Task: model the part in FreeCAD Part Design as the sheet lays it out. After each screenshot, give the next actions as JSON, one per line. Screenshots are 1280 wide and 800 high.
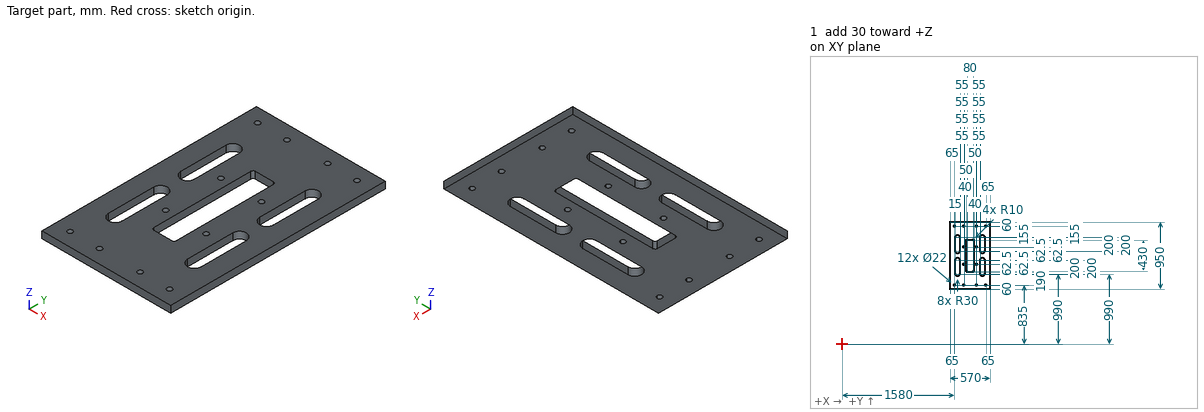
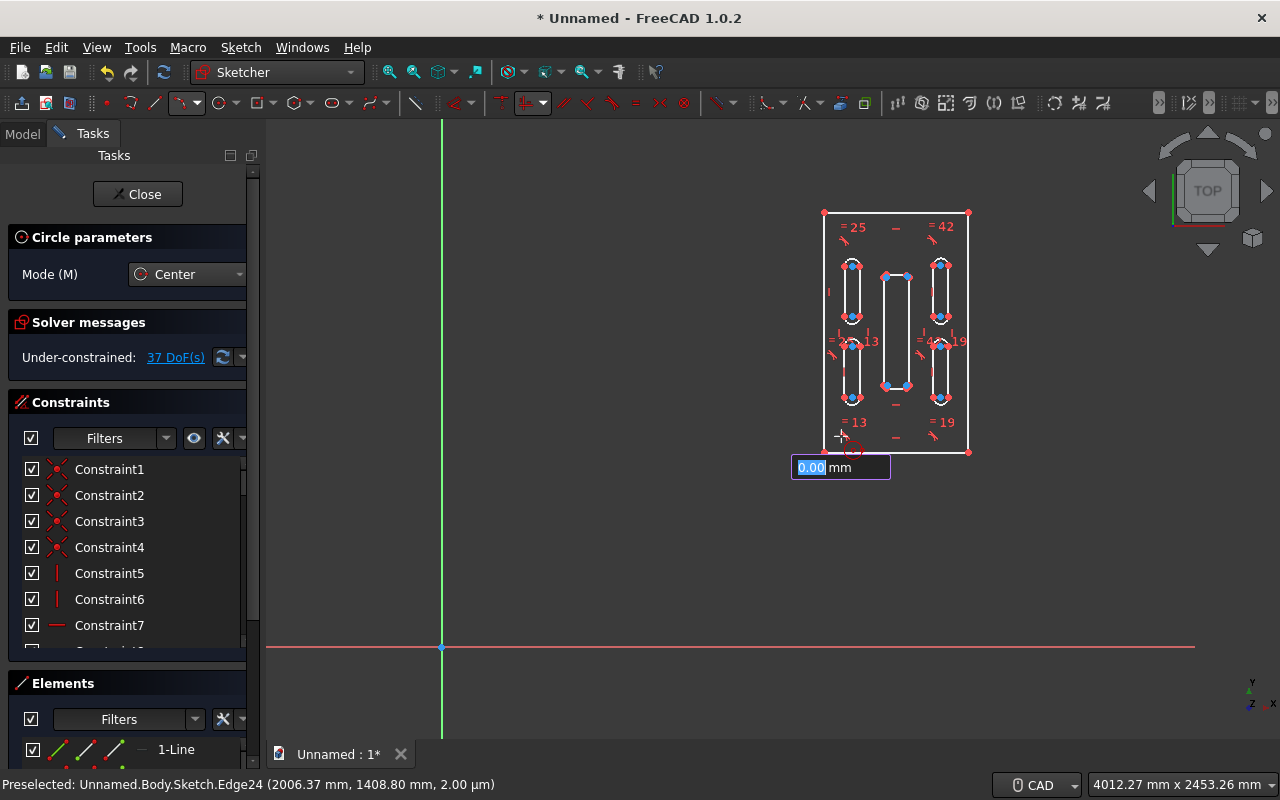
{"action": "scroll", "coordinate": [843, 434], "scroll_direction": "up", "scroll_amount": 9}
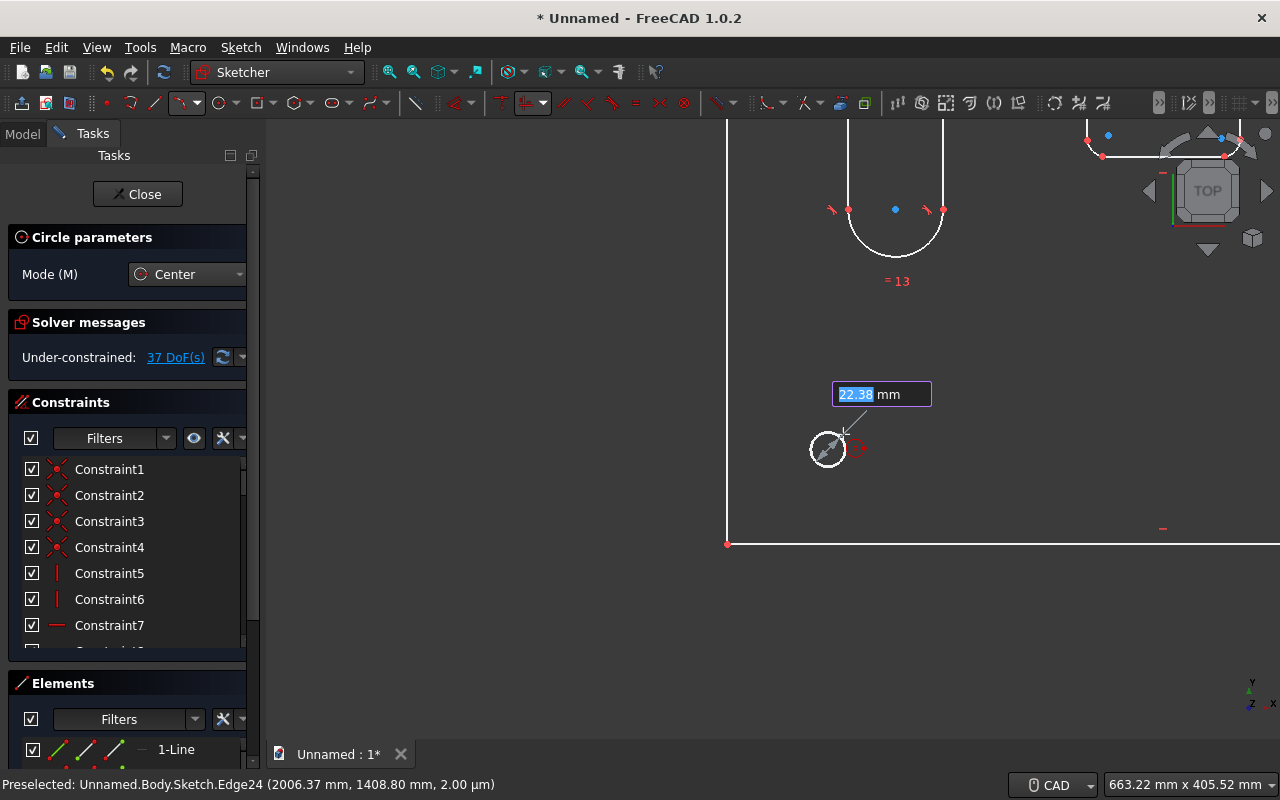
{"action": "left_click", "coordinate": [840, 433]}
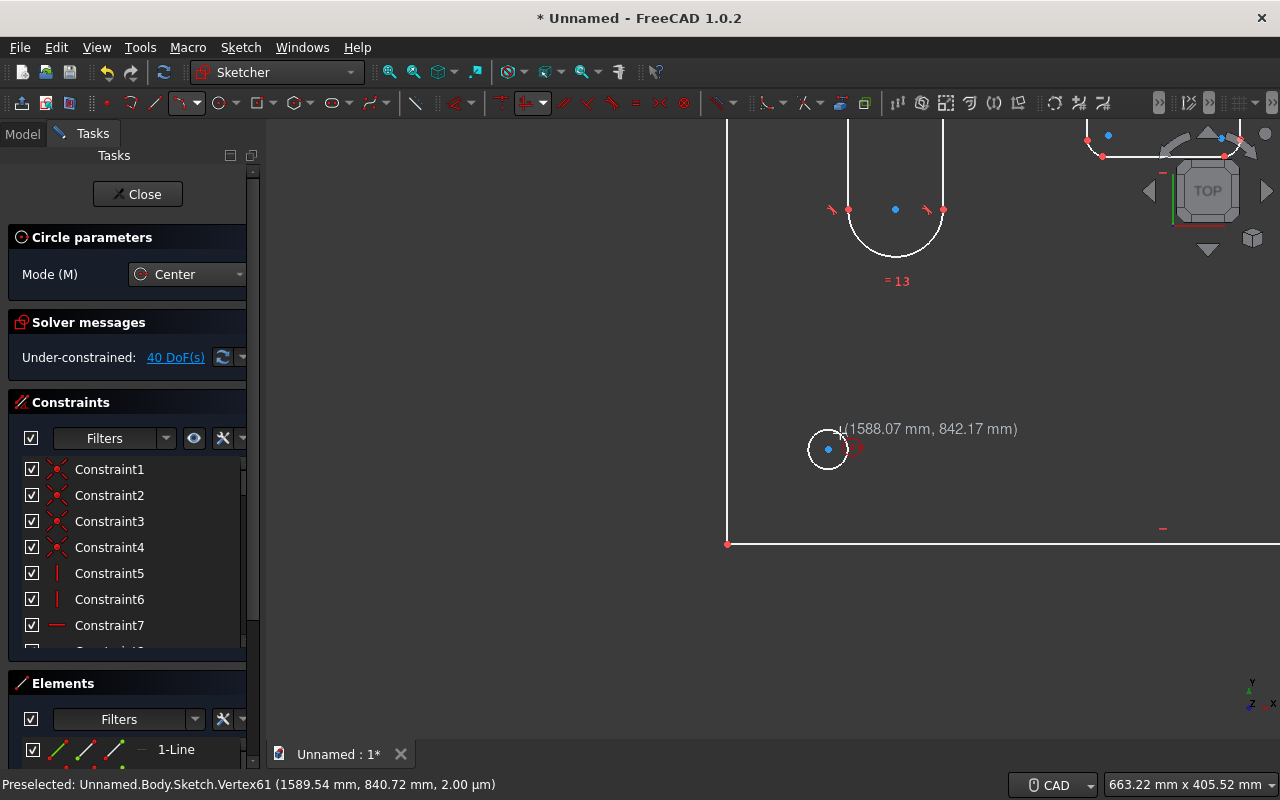
{"action": "scroll", "coordinate": [1026, 445], "scroll_direction": "up", "scroll_amount": 2}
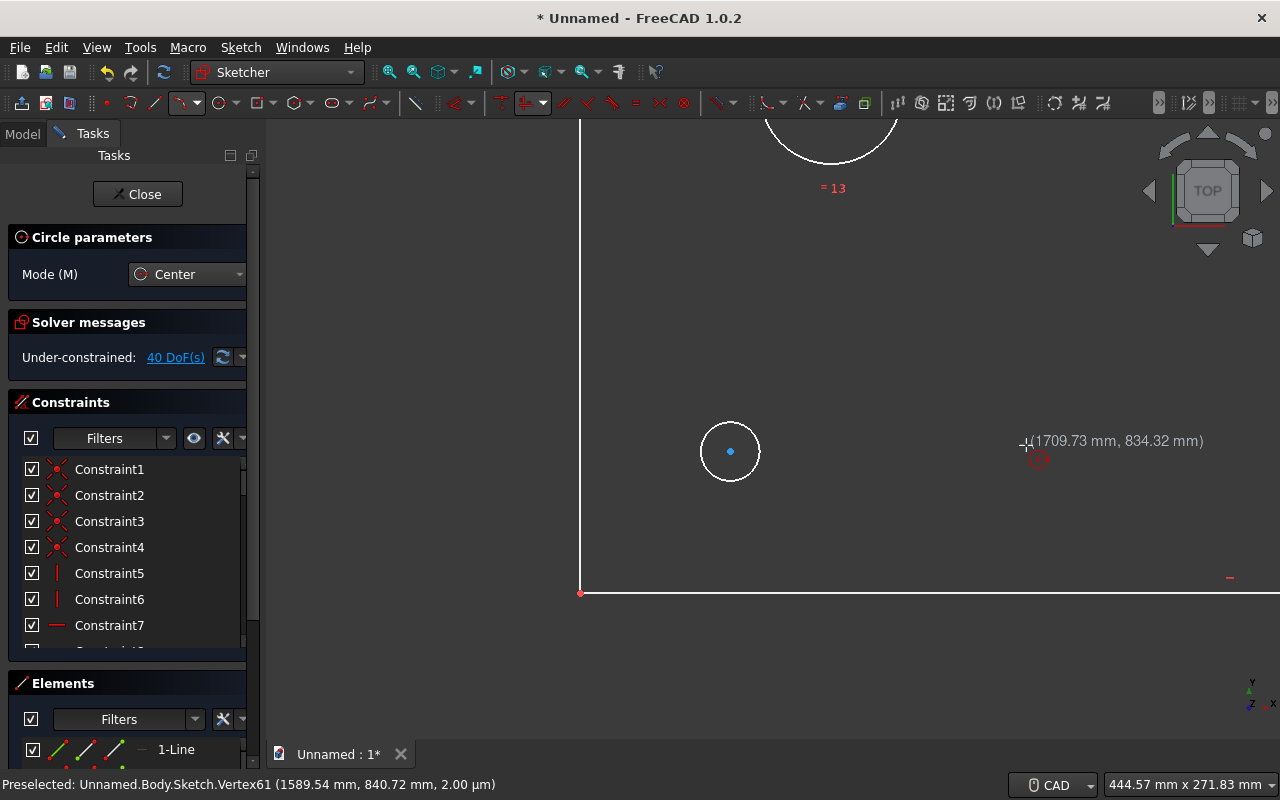
{"action": "scroll", "coordinate": [854, 435], "scroll_direction": "down", "scroll_amount": 11}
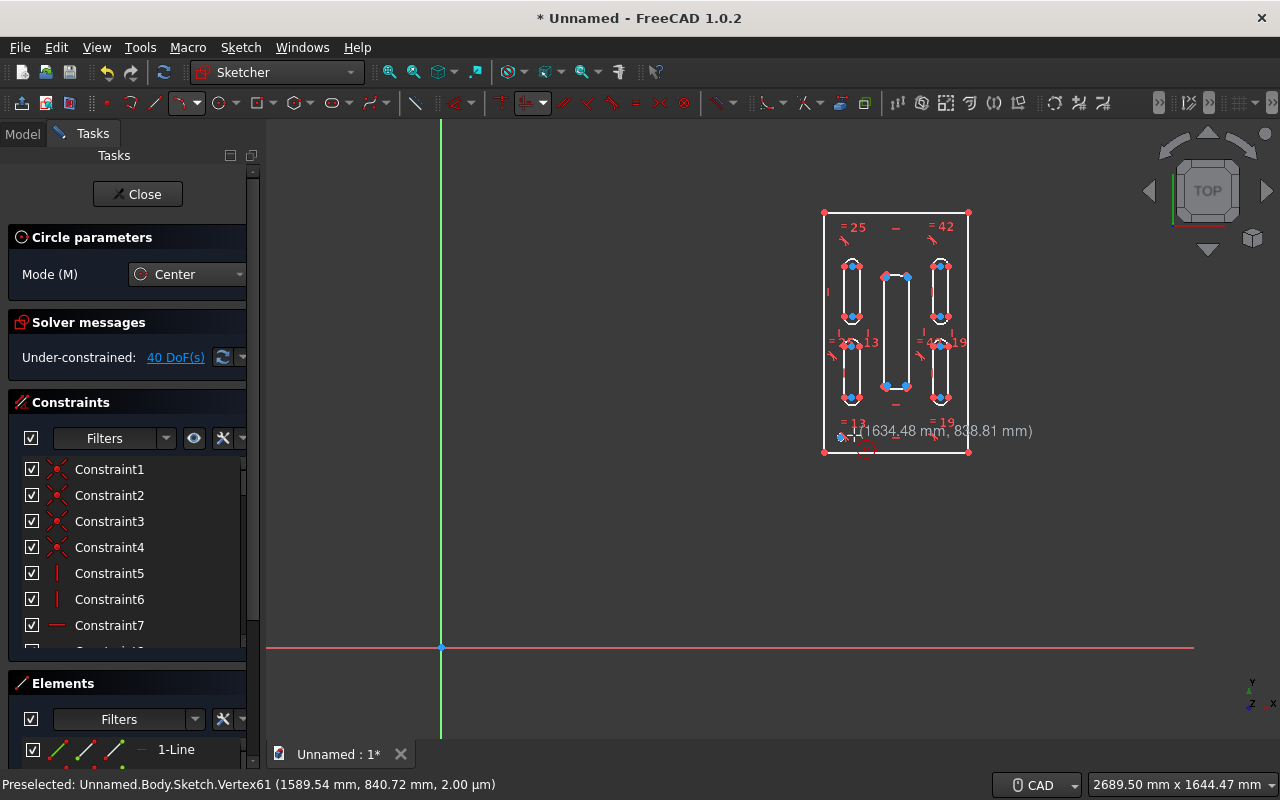
{"action": "left_click", "coordinate": [874, 437]}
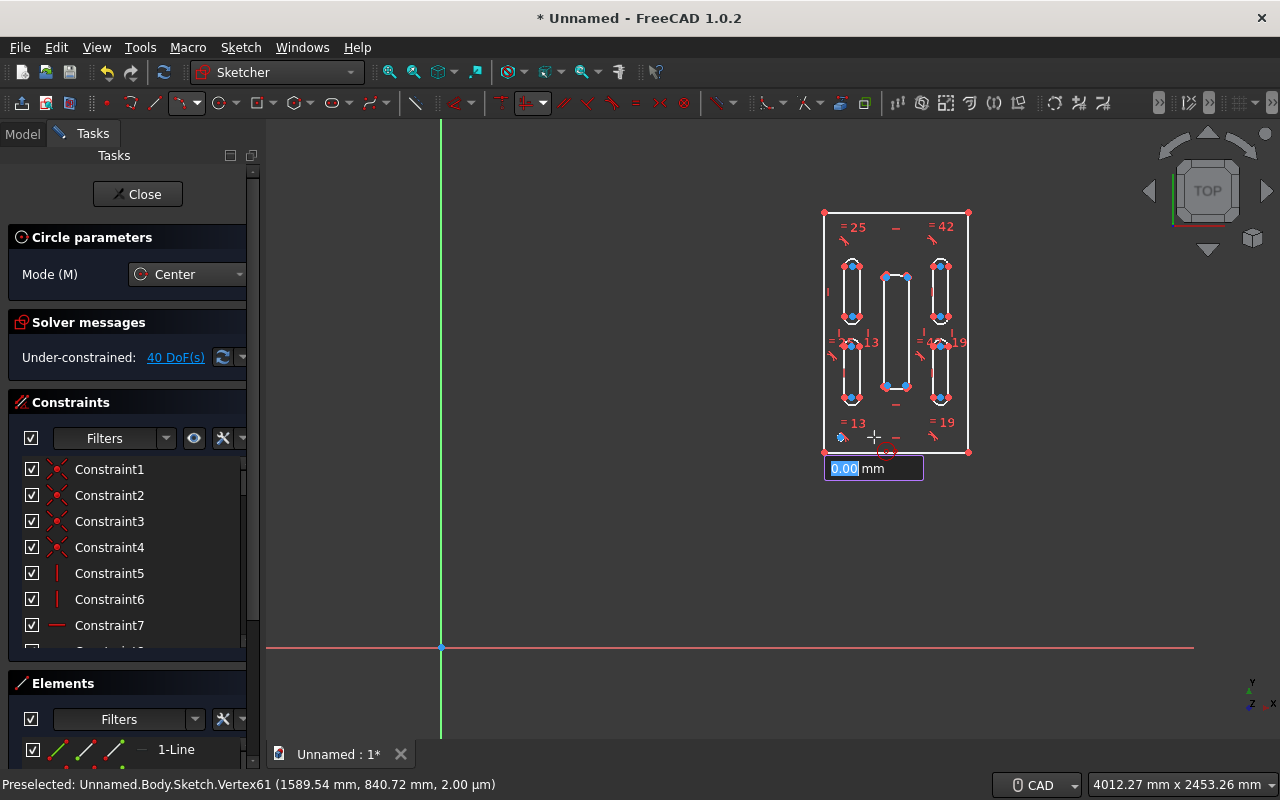
{"action": "scroll", "coordinate": [876, 435], "scroll_direction": "up", "scroll_amount": 9}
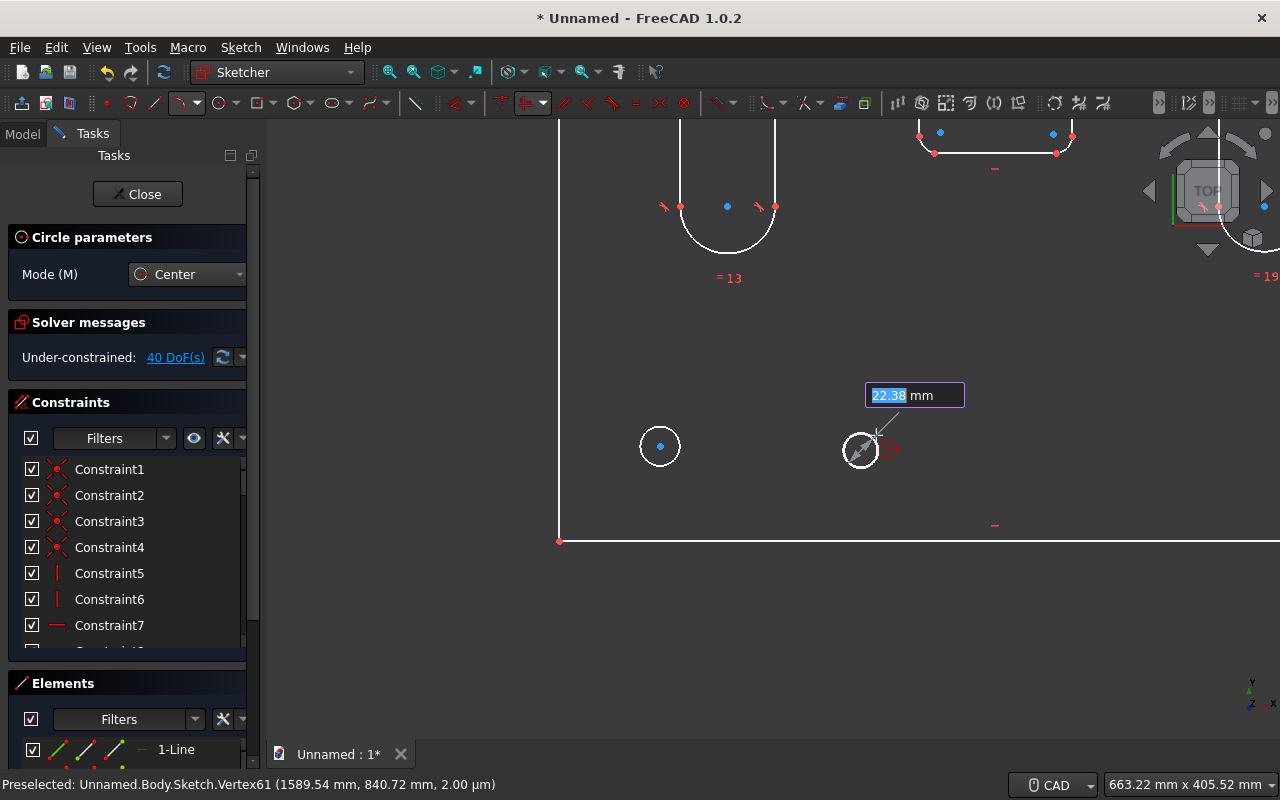
{"action": "left_click", "coordinate": [870, 430]}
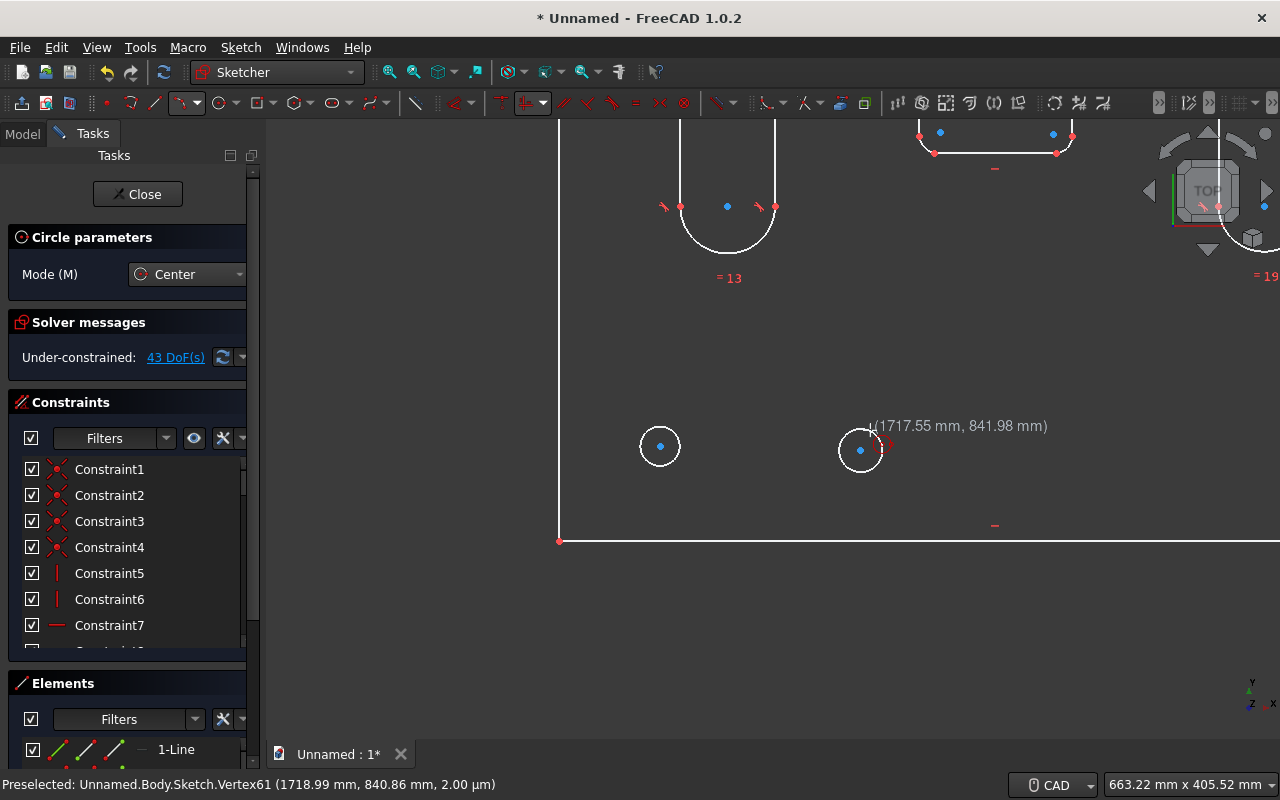
{"action": "scroll", "coordinate": [876, 435], "scroll_direction": "down", "scroll_amount": 9}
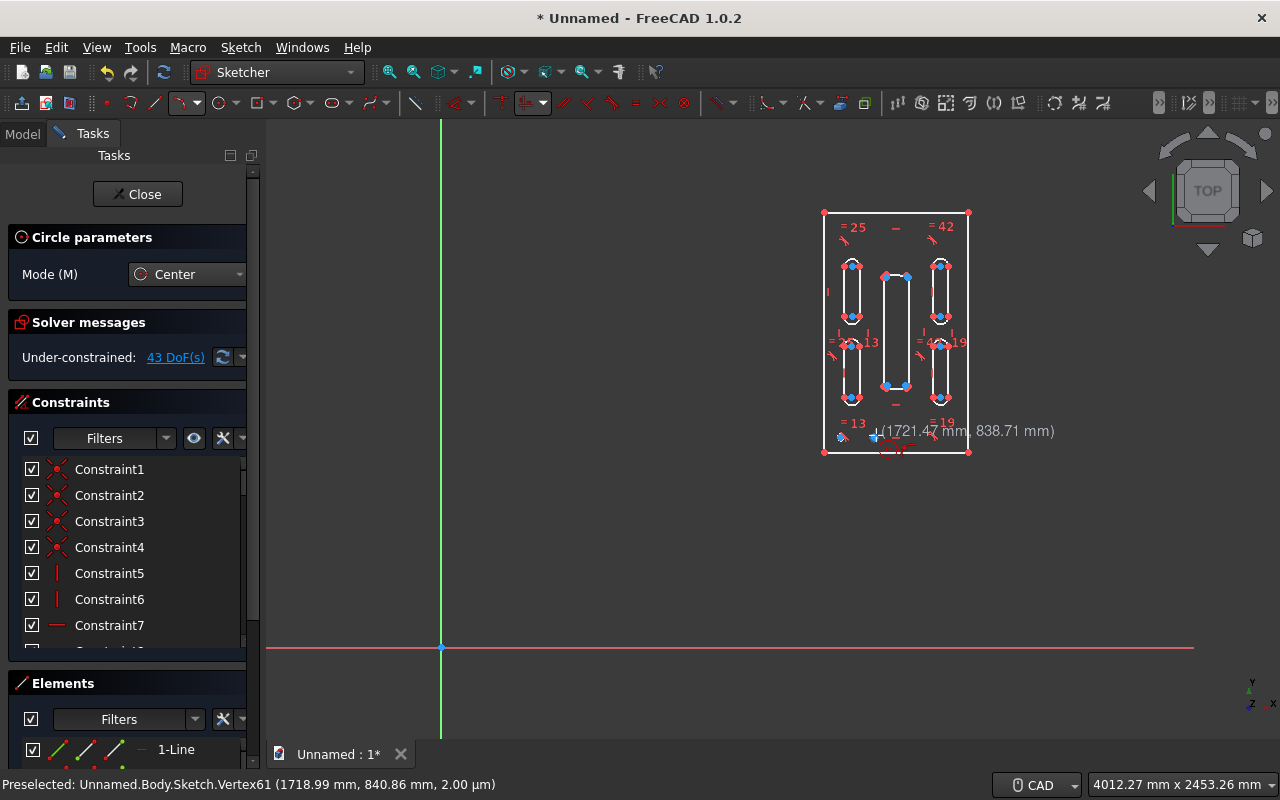
{"action": "scroll", "coordinate": [874, 363], "scroll_direction": "up", "scroll_amount": 11}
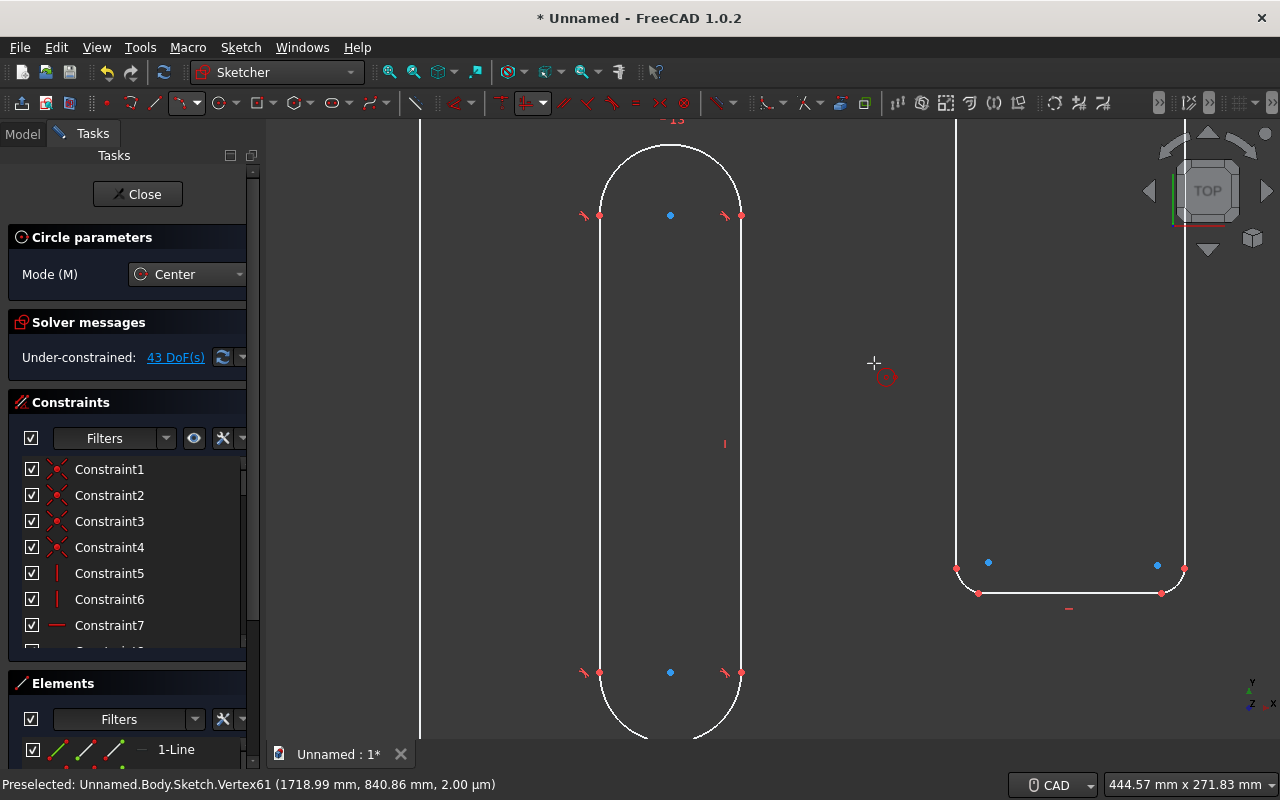
{"action": "scroll", "coordinate": [874, 363], "scroll_direction": "down", "scroll_amount": 11}